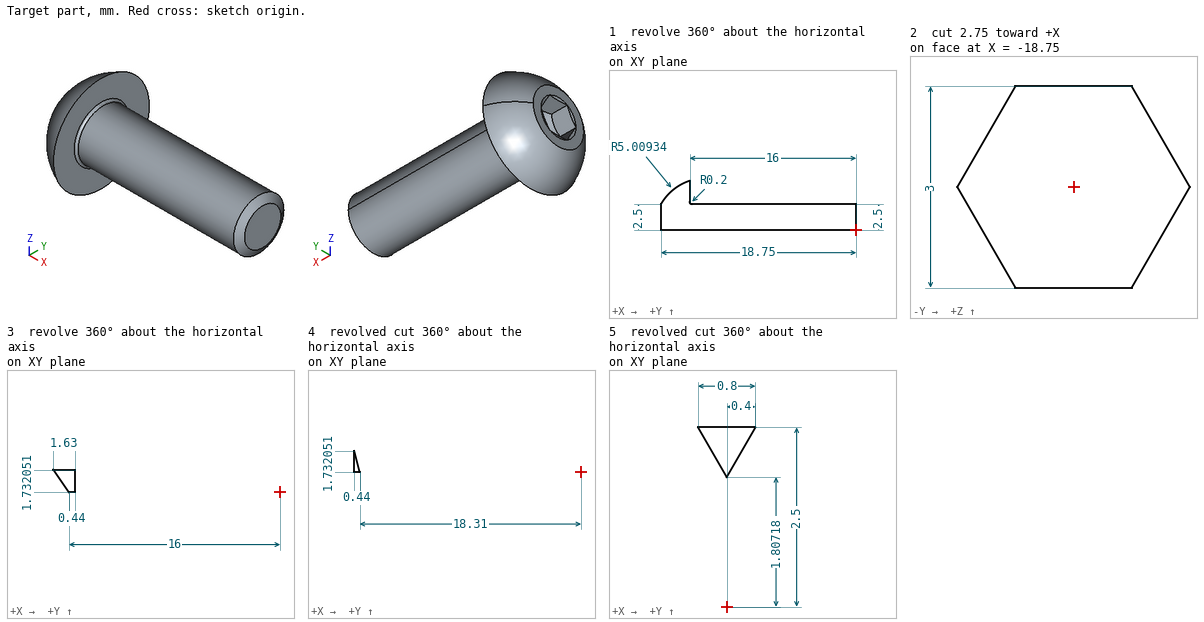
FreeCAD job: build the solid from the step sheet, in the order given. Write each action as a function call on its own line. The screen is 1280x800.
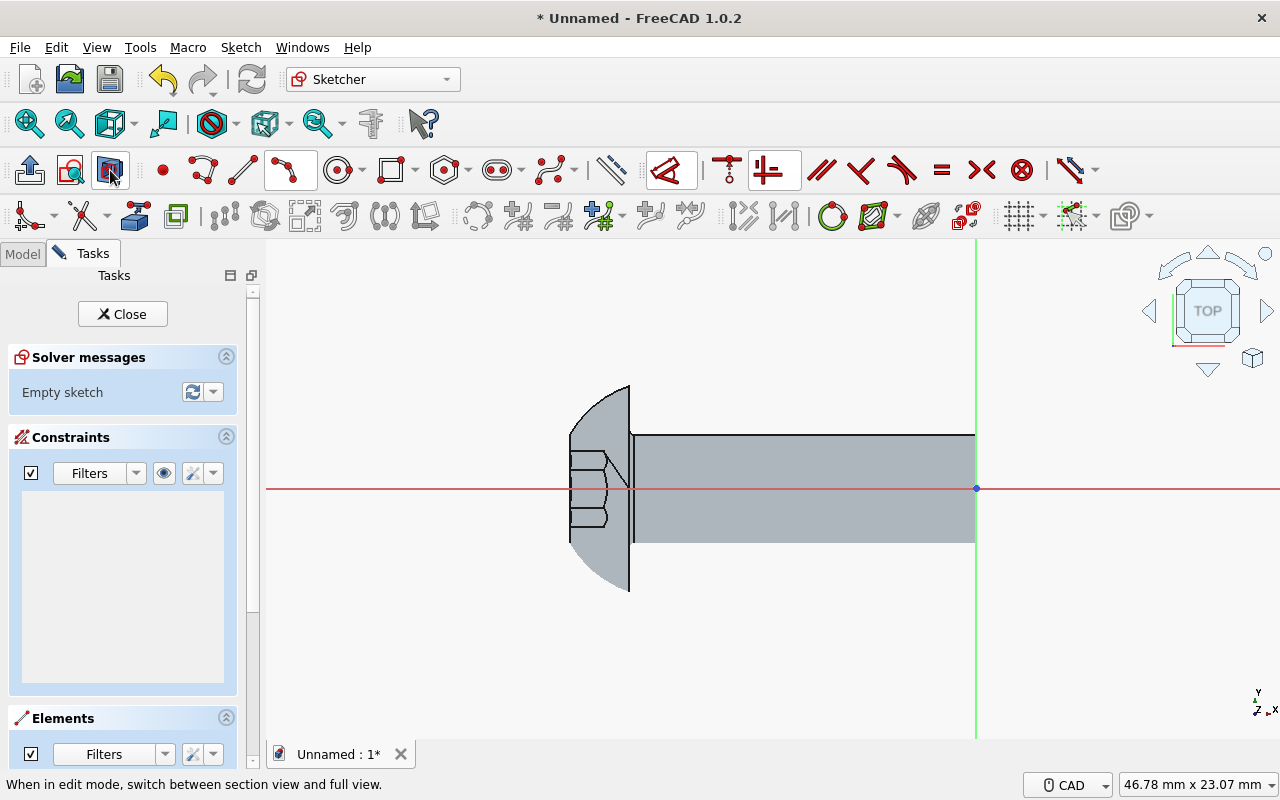
scroll(990, 440, up, 15)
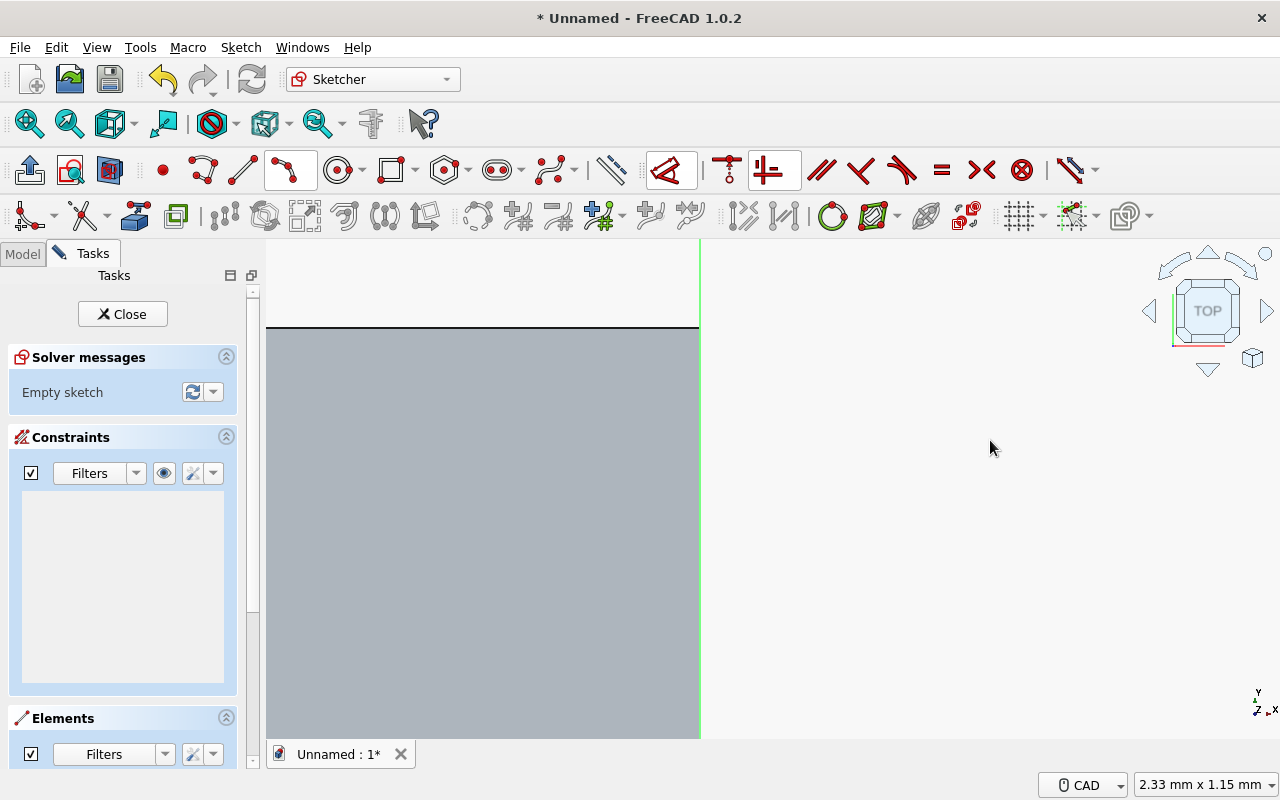
click(204, 170)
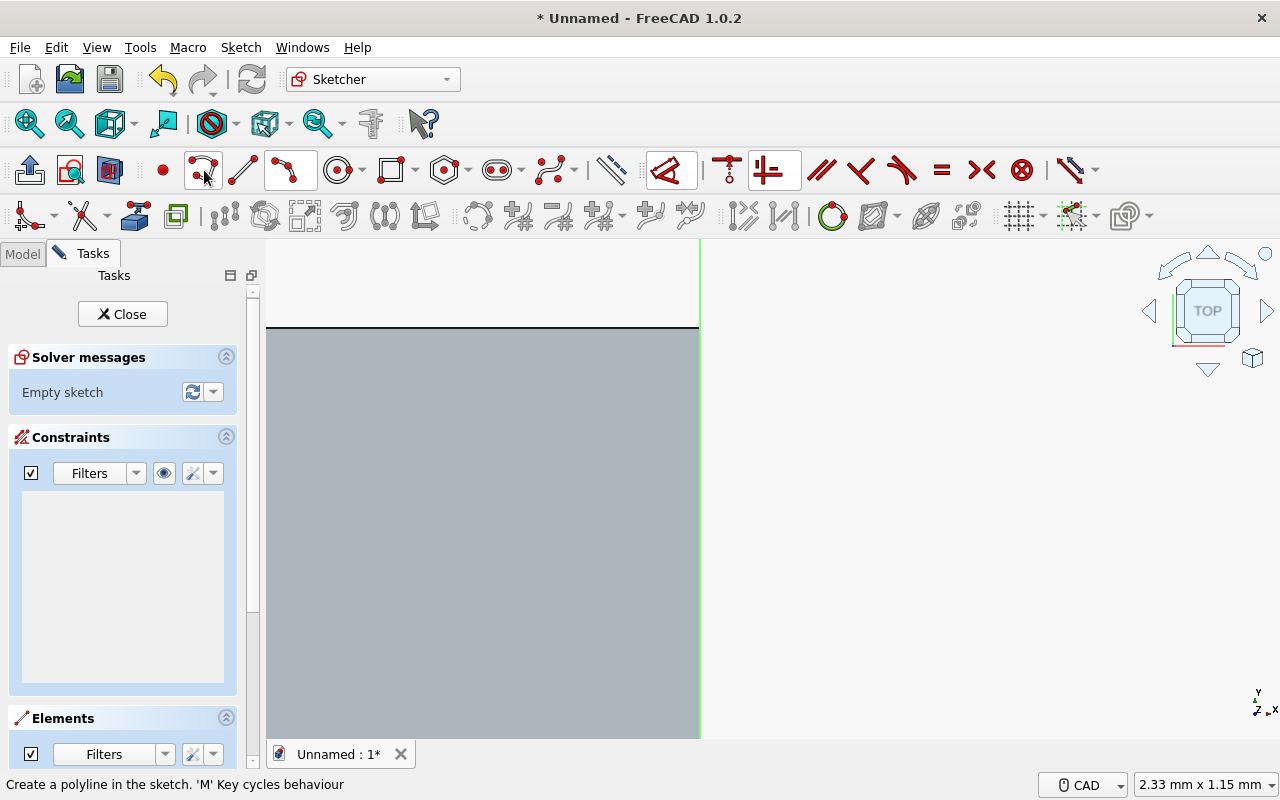
click(700, 630)
click(874, 328)
click(525, 328)
click(700, 631)
key(Escape)
key(Escape)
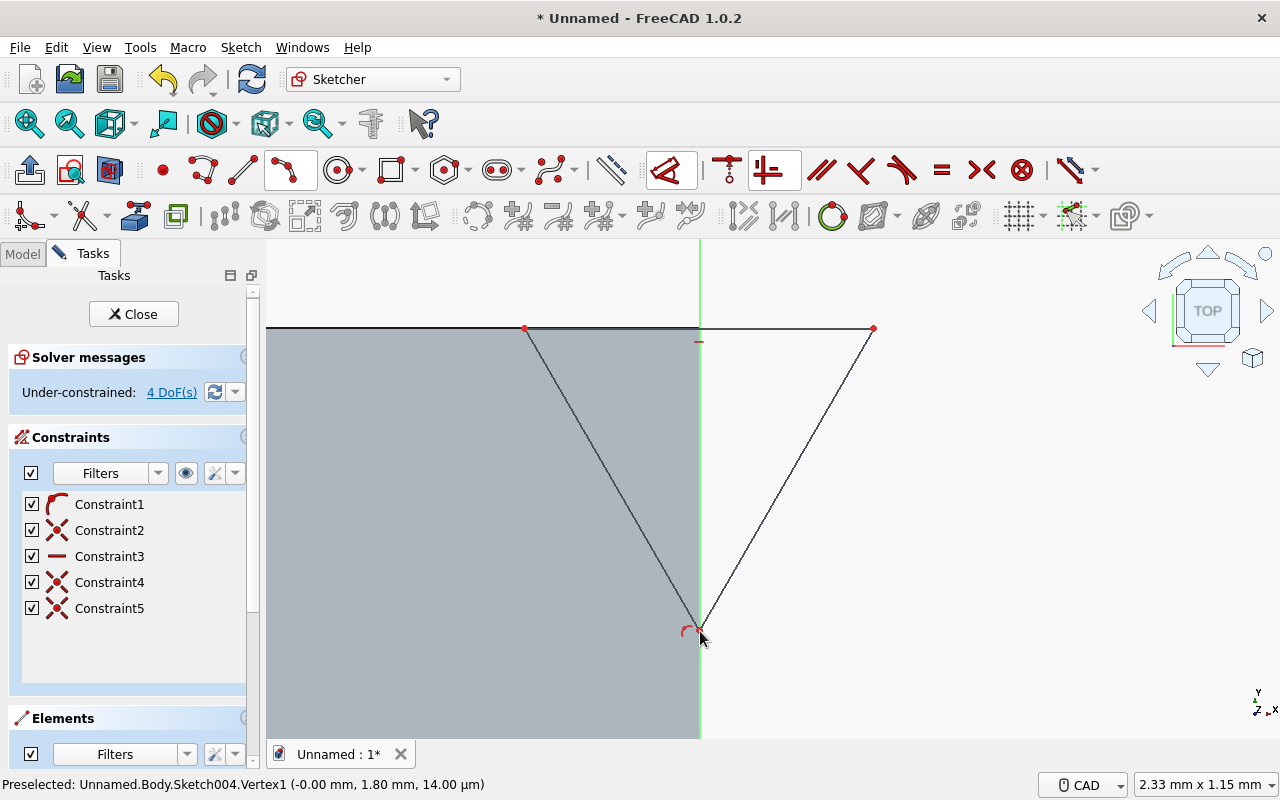
click(769, 329)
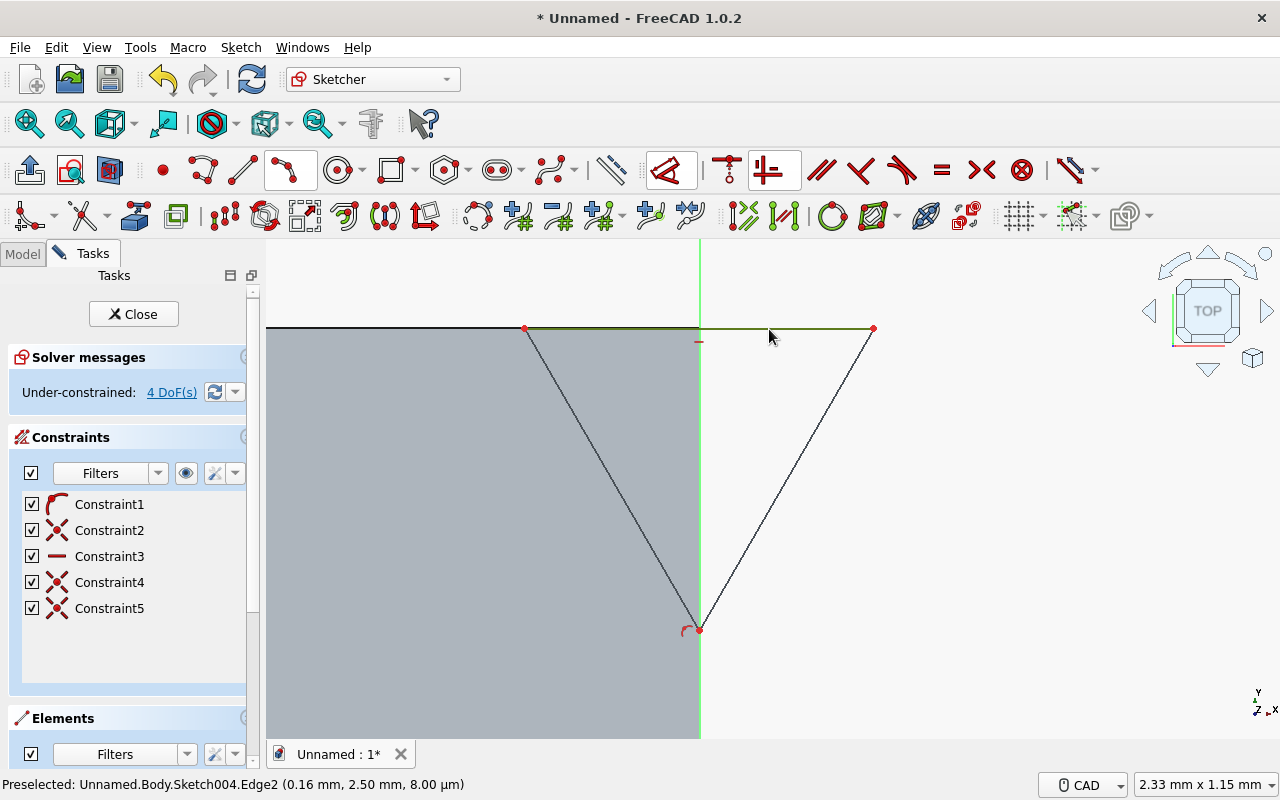
click(692, 170)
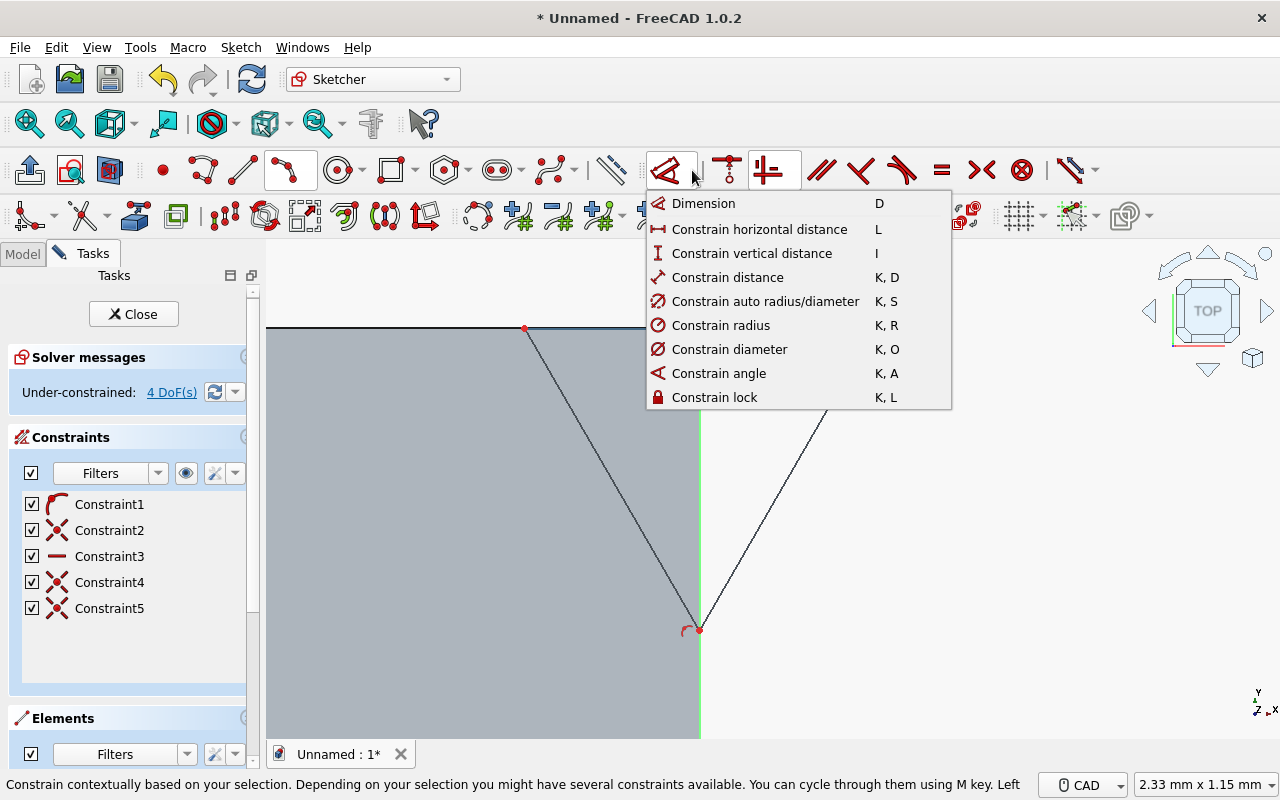
click(799, 229)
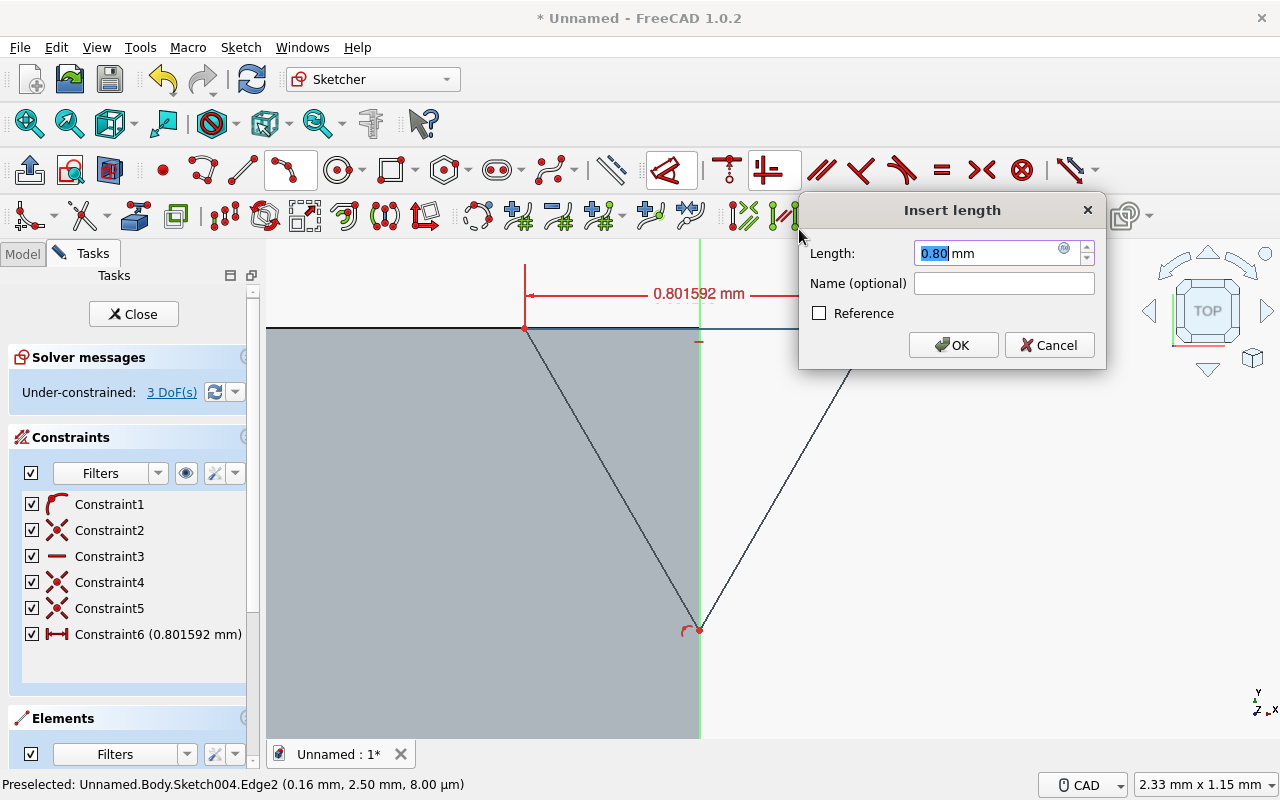
text(0.8)
key(Return)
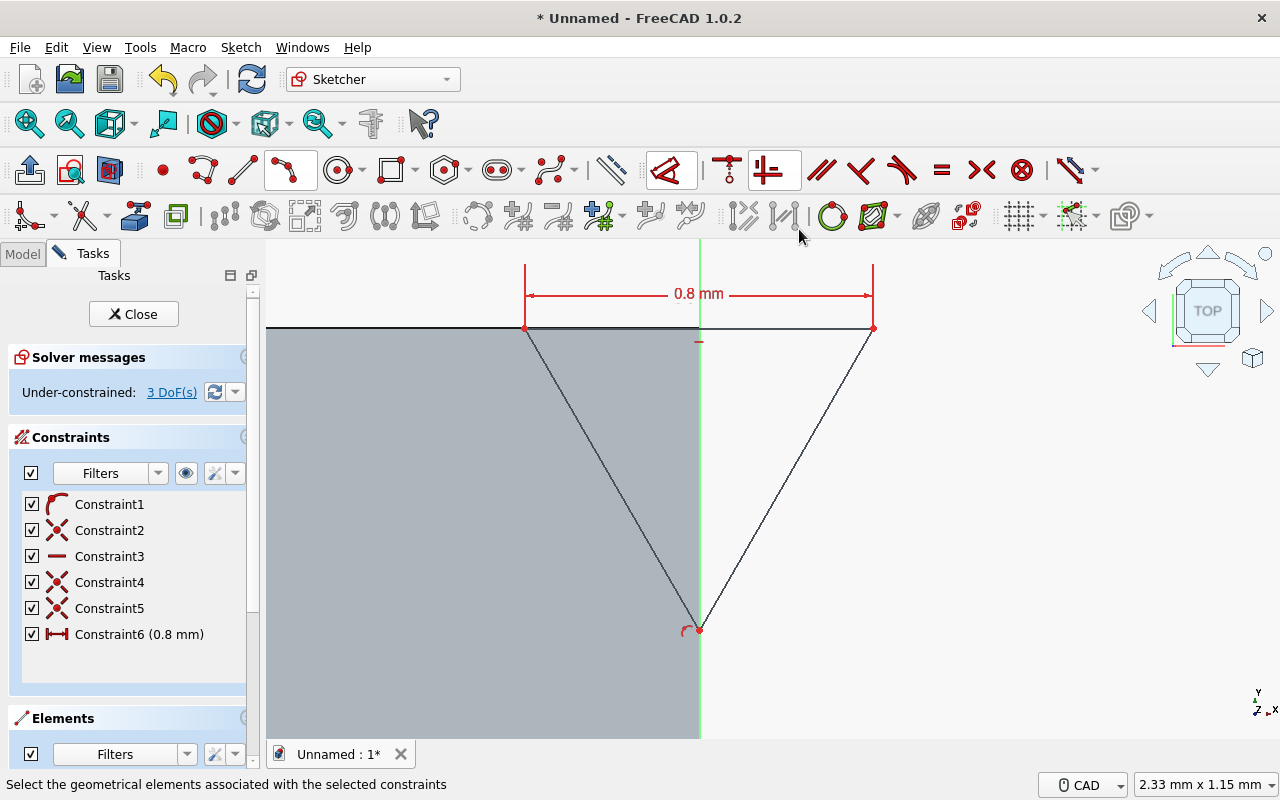
click(873, 329)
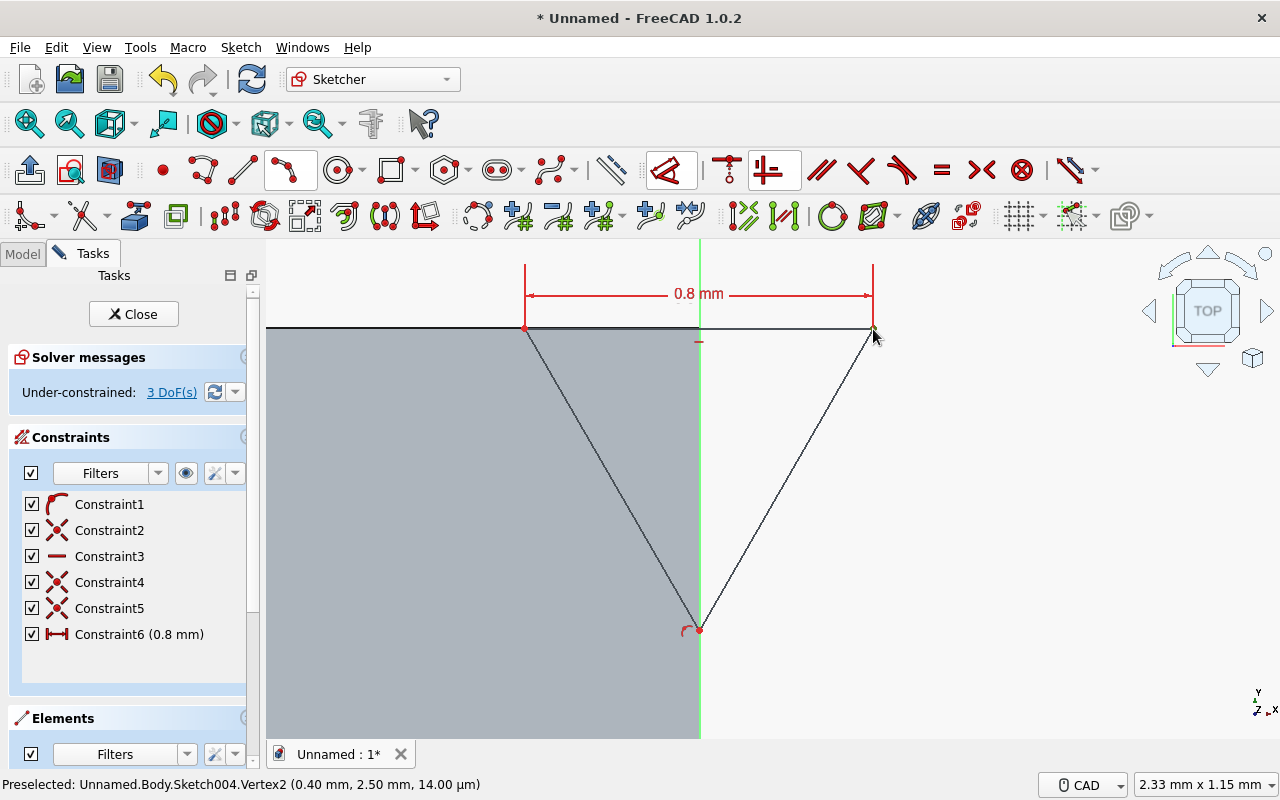
key(l)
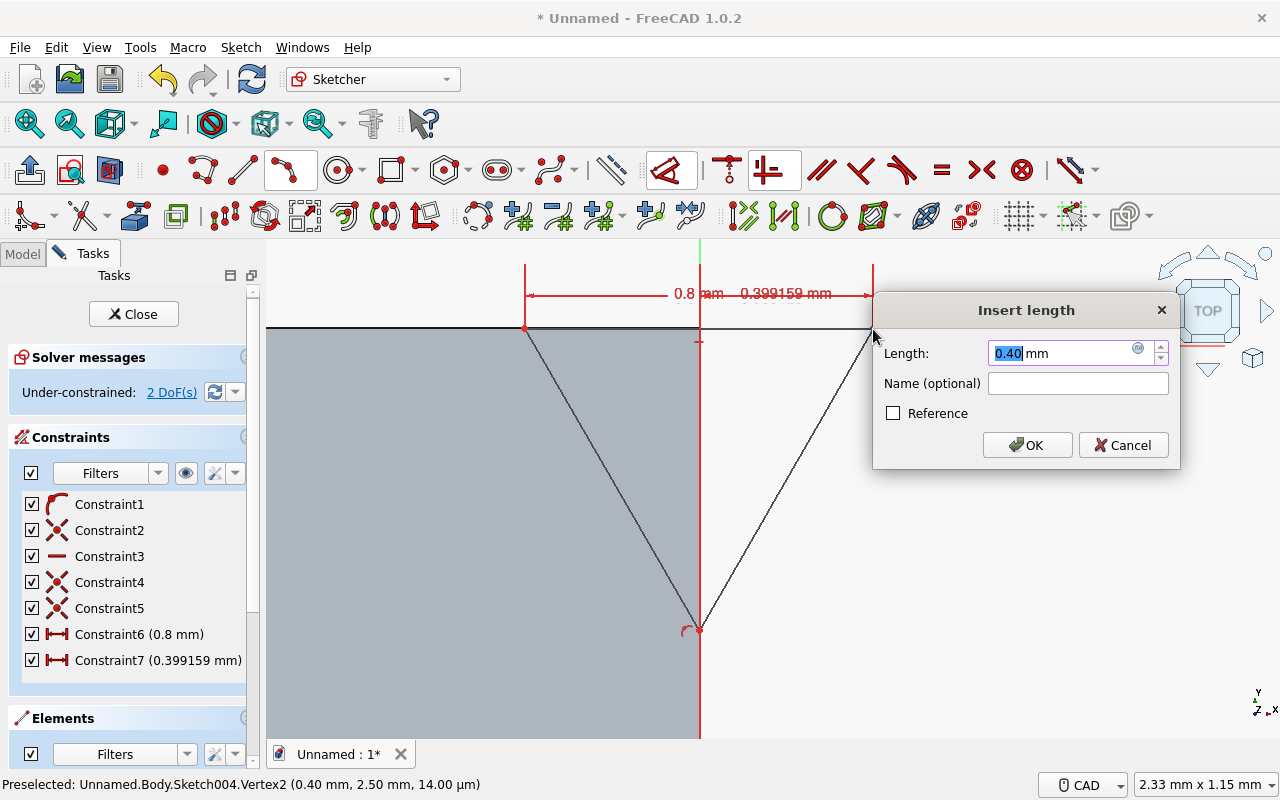
text(0.4)
key(Return)